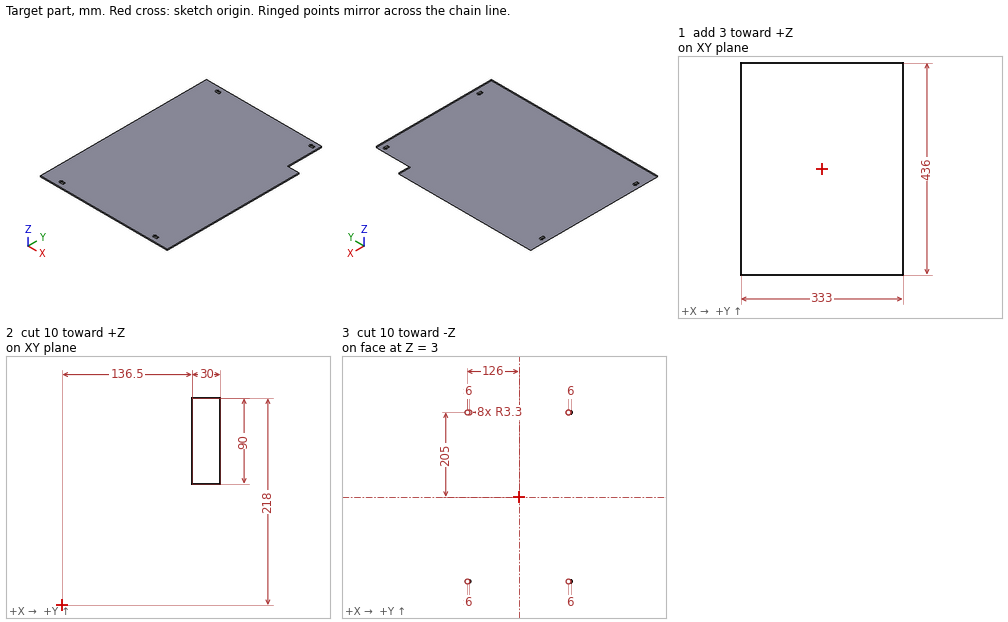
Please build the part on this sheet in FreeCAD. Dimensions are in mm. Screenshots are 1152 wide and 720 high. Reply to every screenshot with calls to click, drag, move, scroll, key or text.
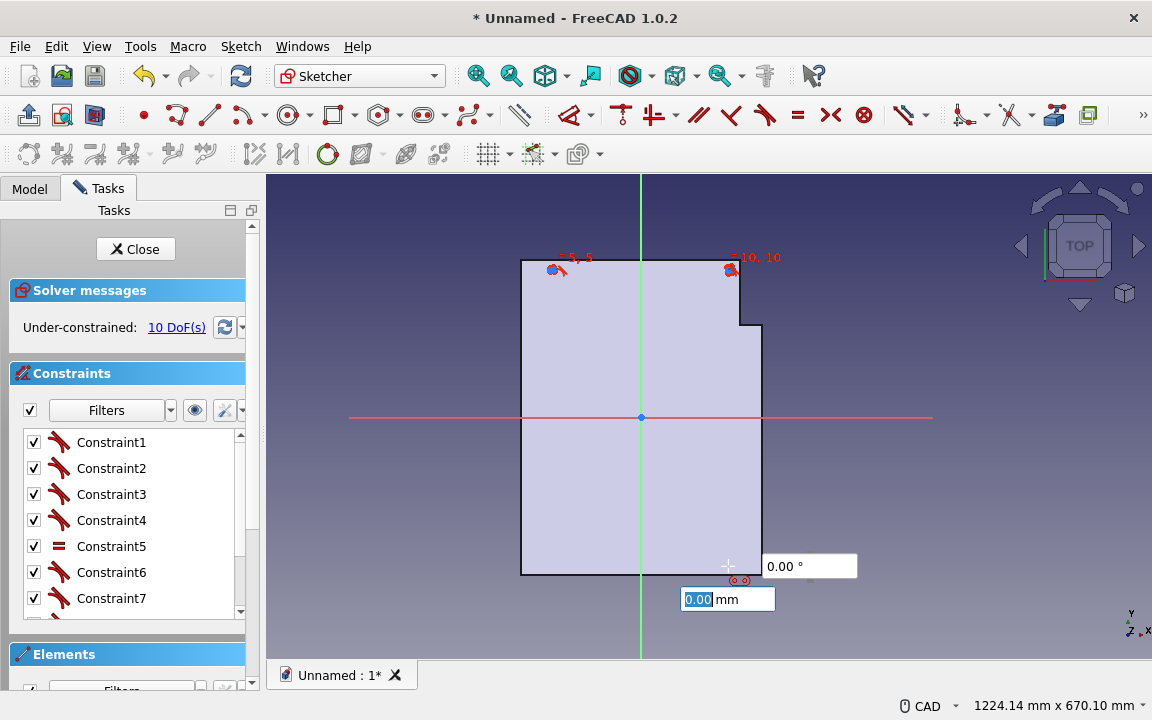
scroll(732, 566, up, 7)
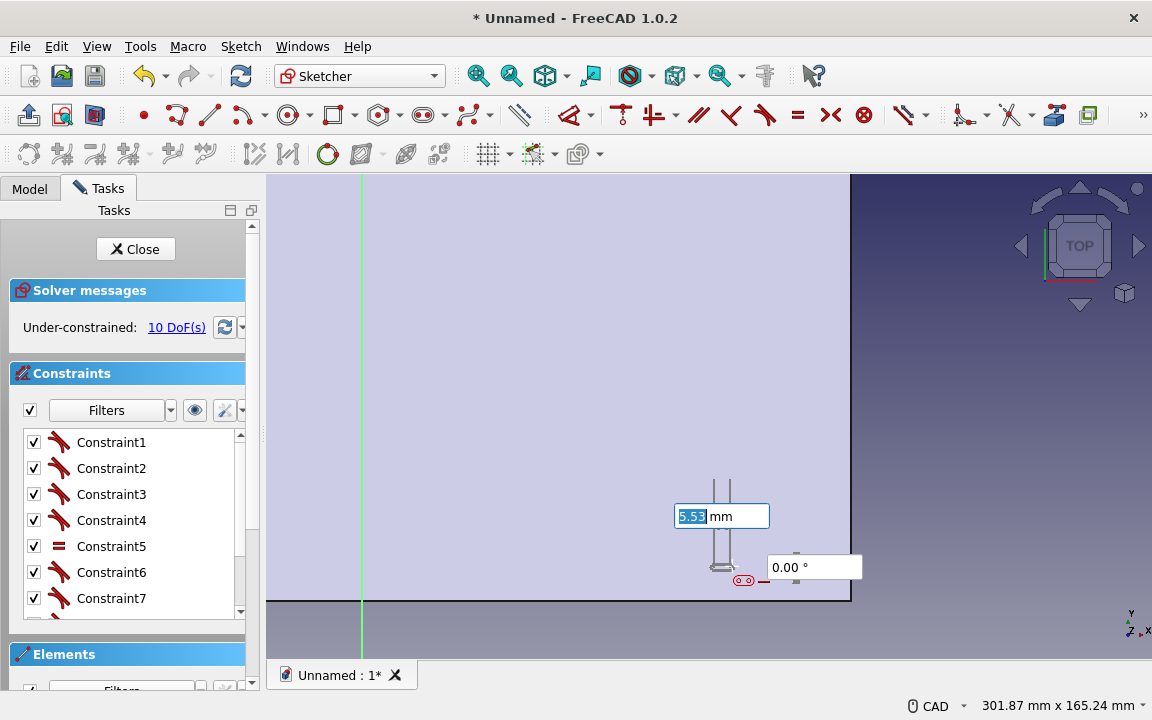
click(732, 564)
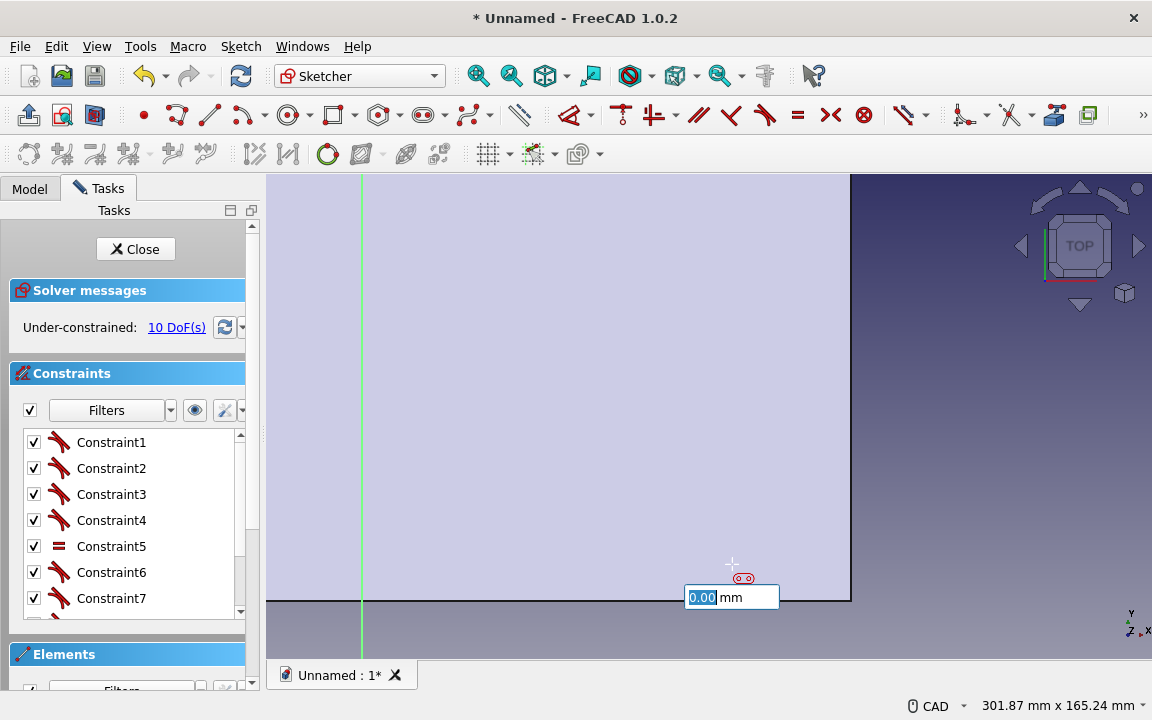
scroll(723, 554, up, 3)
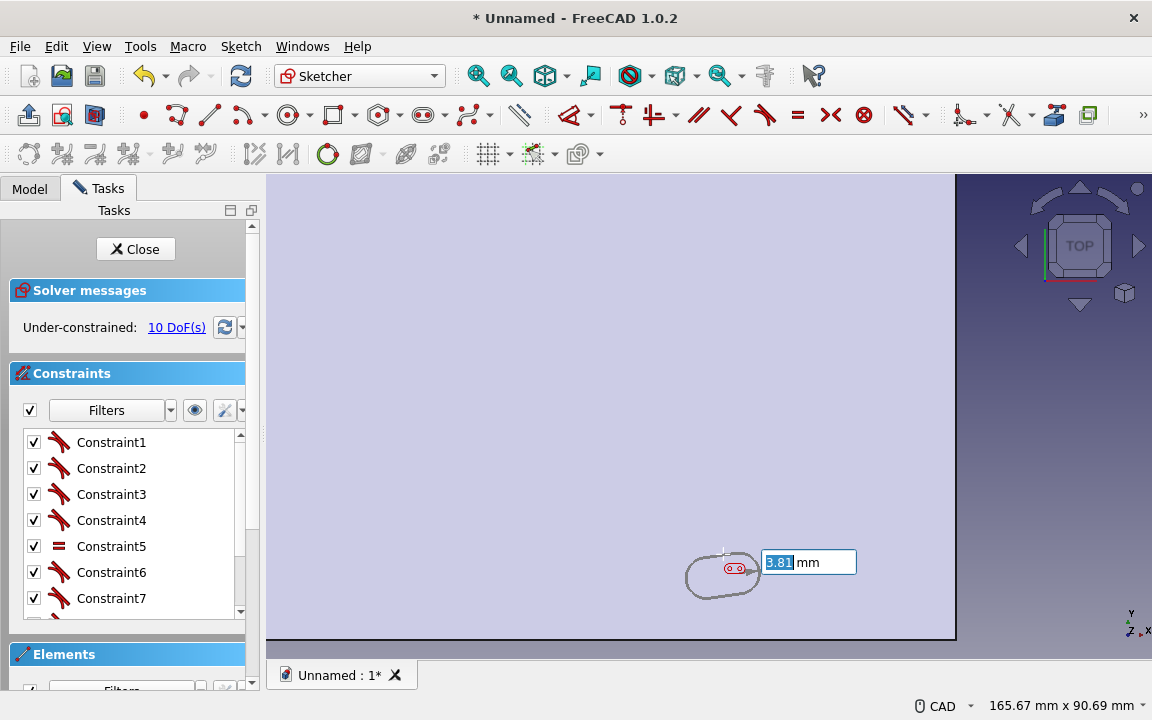
click(723, 553)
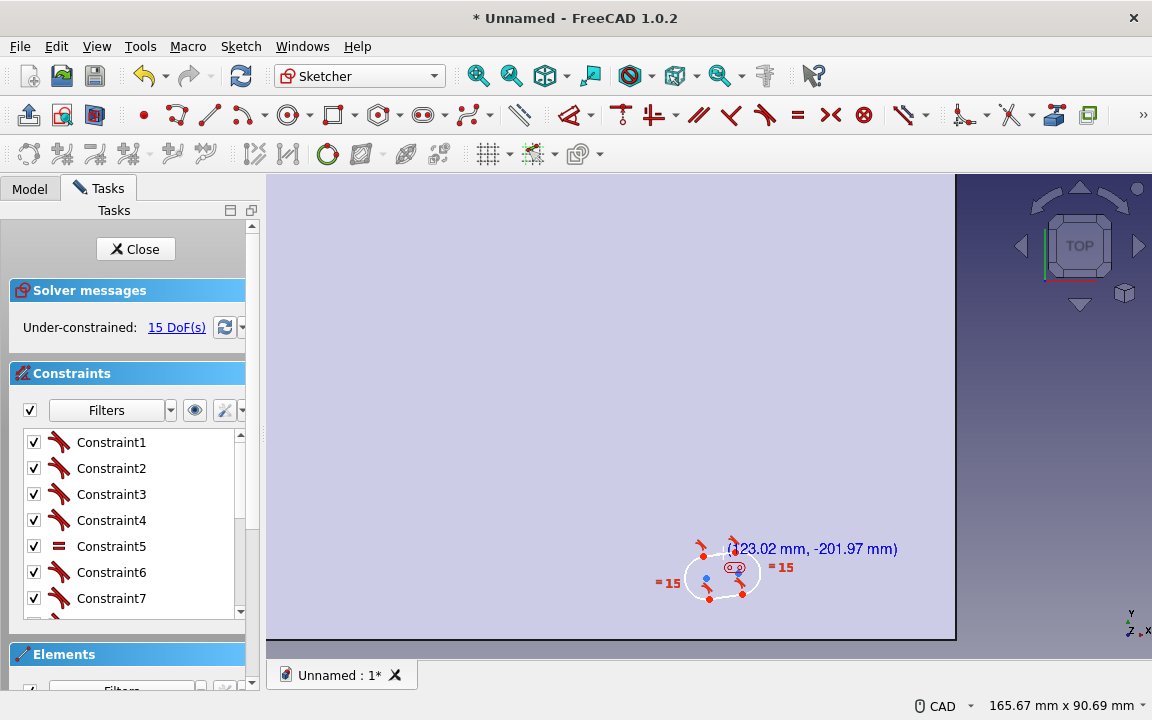
scroll(731, 564, down, 10)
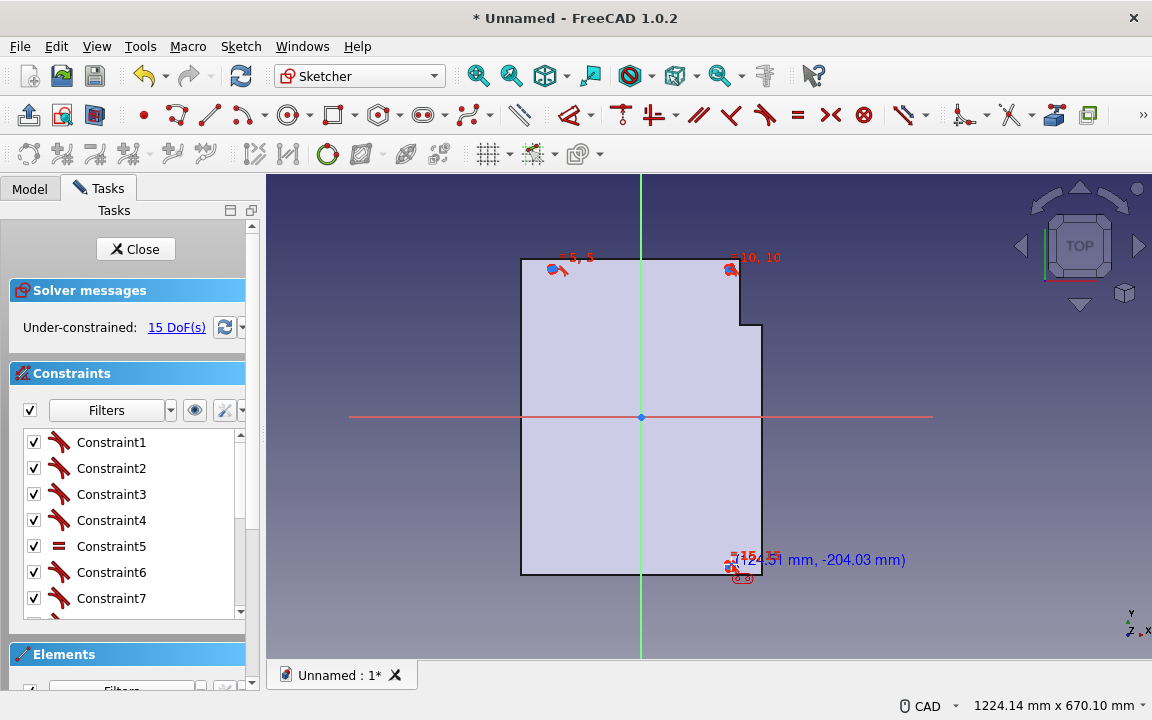
scroll(550, 566, up, 12)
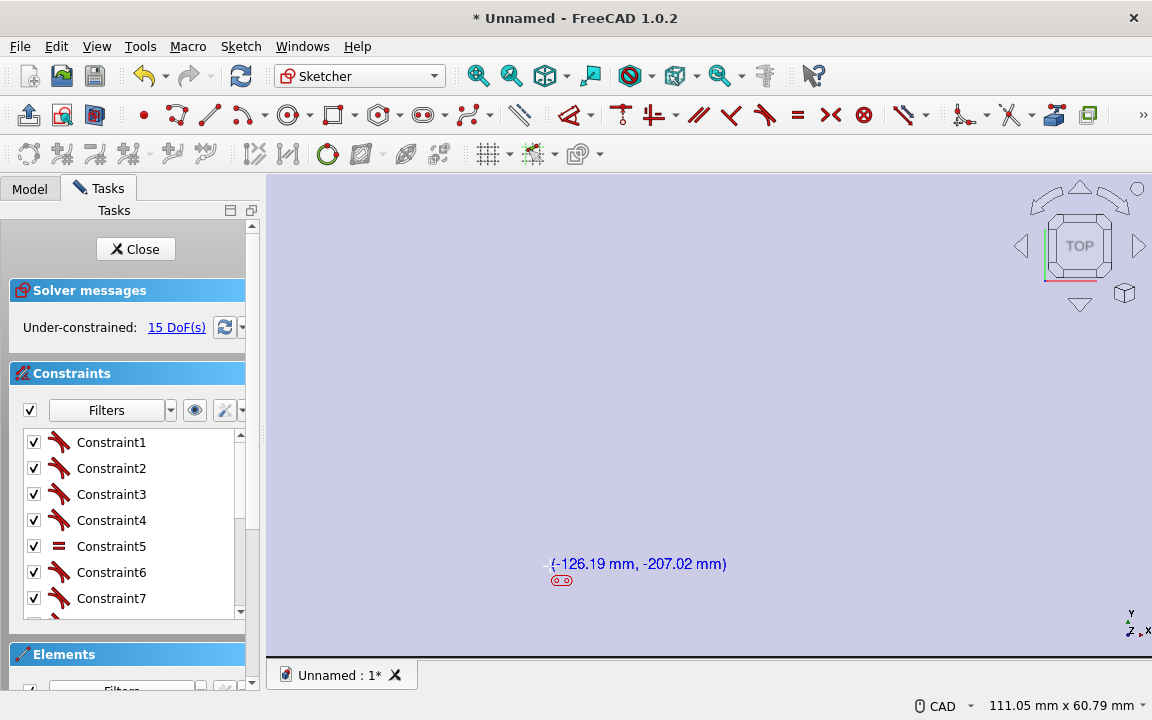
scroll(549, 566, down, 12)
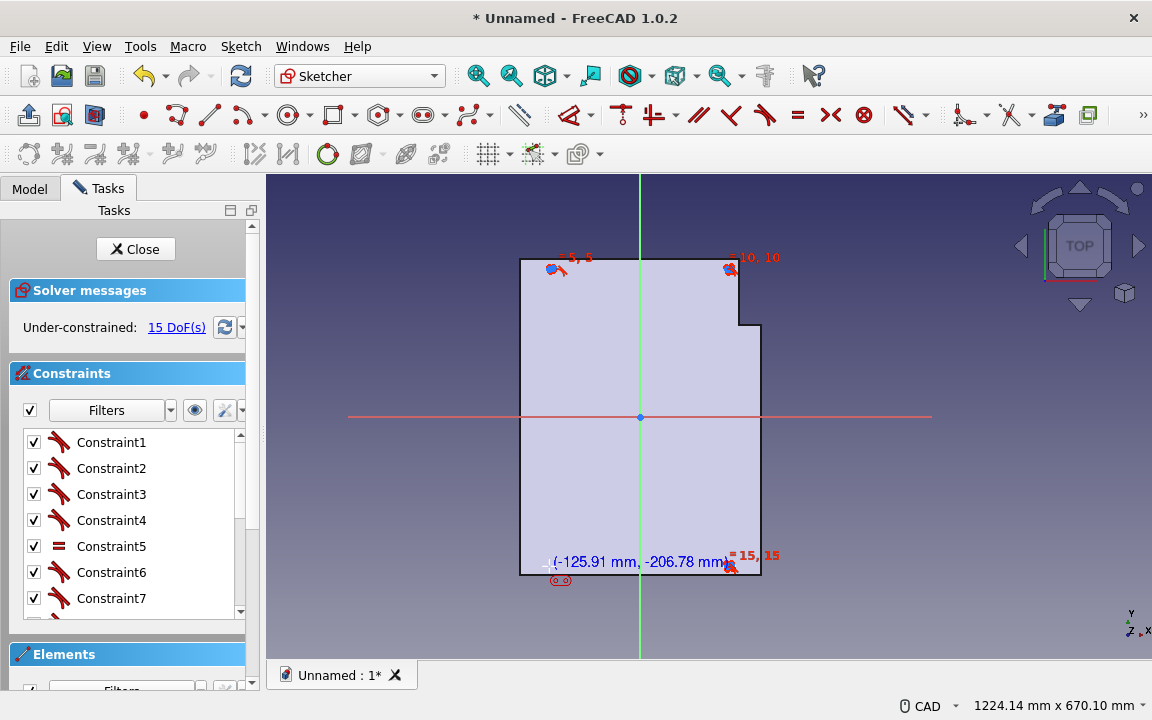
click(549, 566)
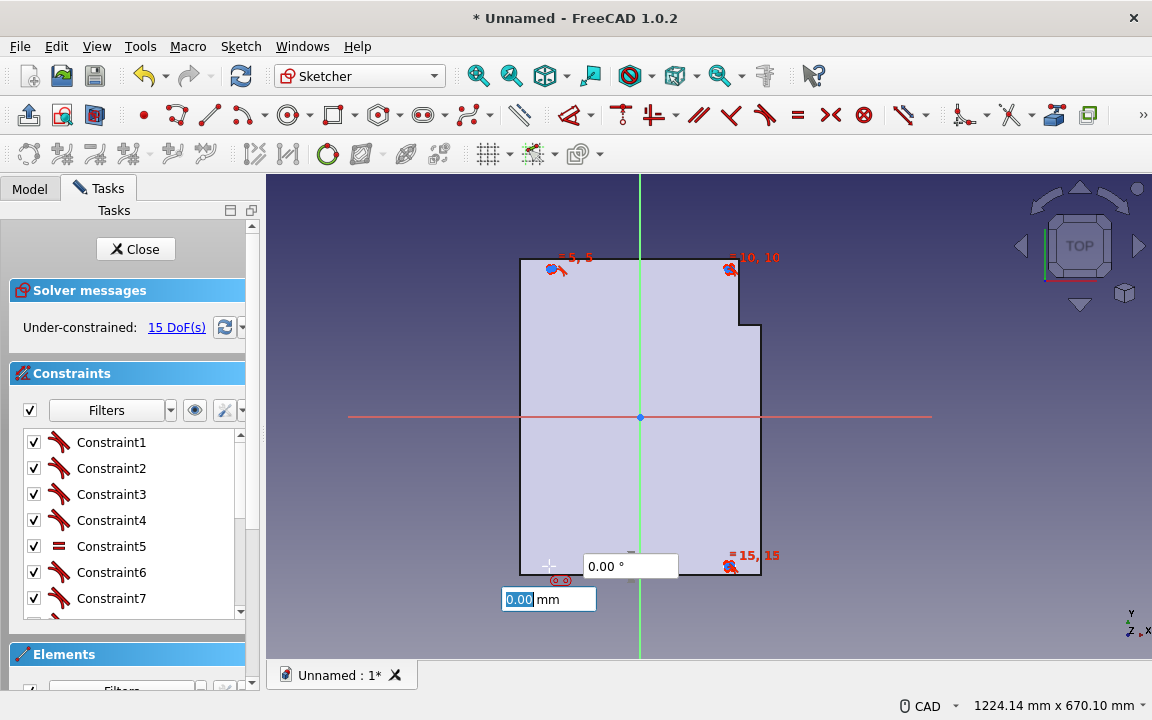
scroll(554, 566, up, 7)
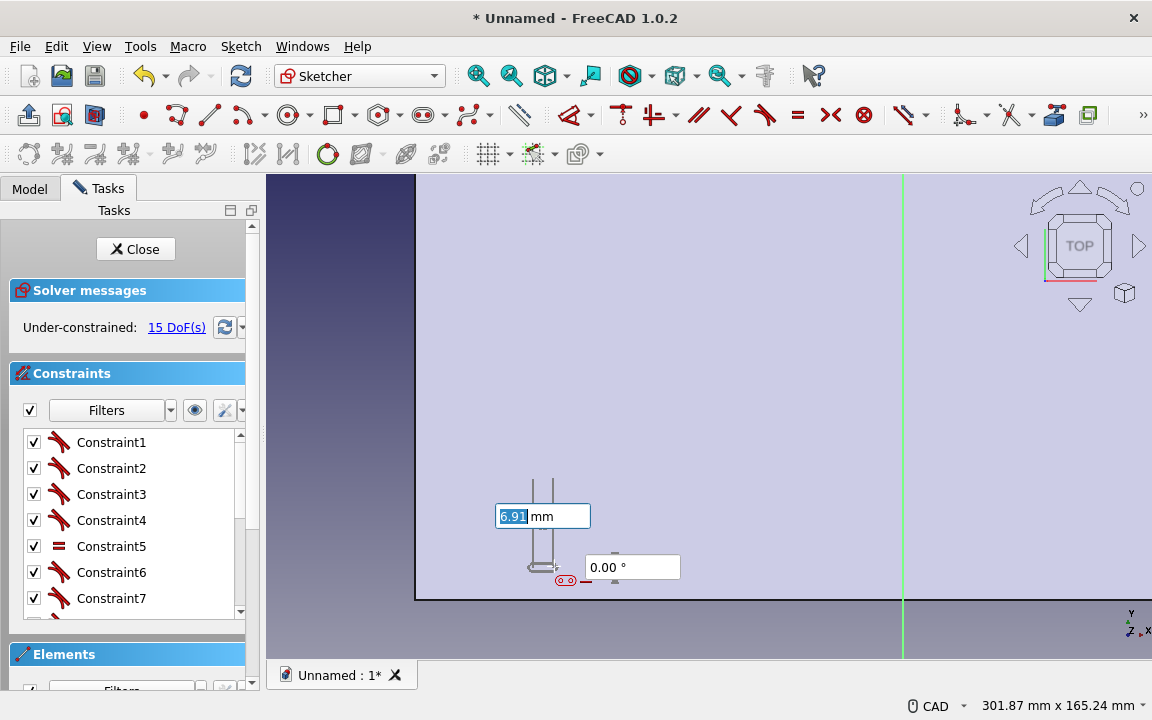
click(551, 564)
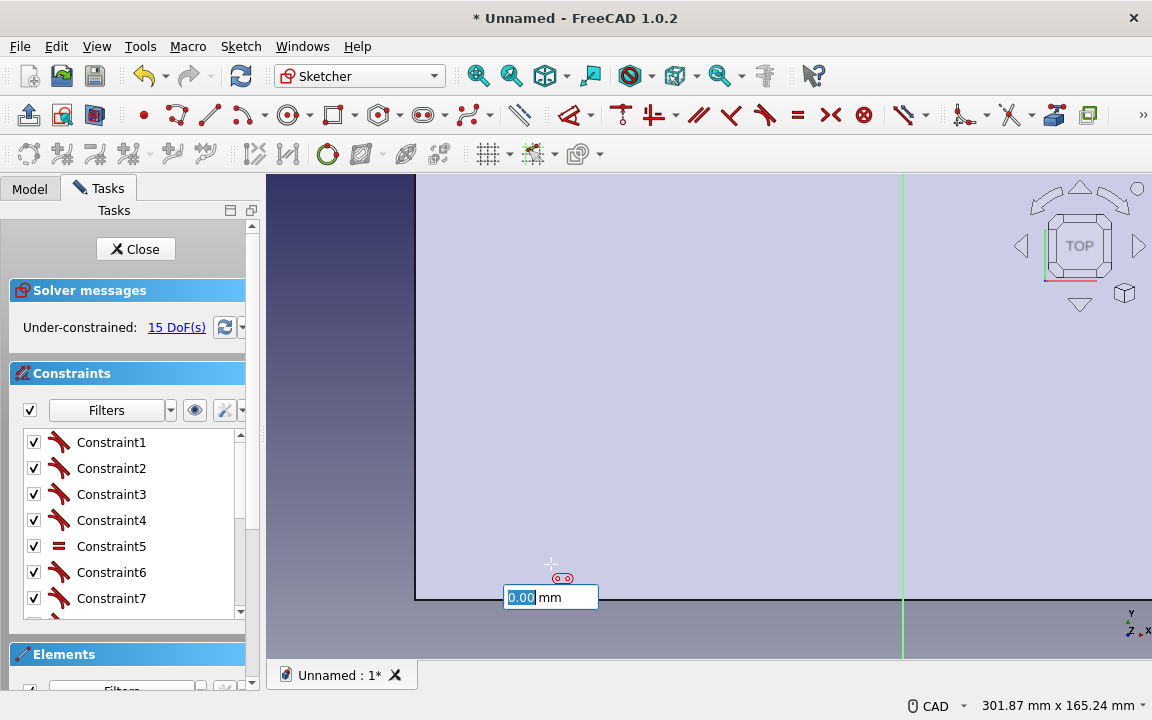
scroll(542, 571, up, 3)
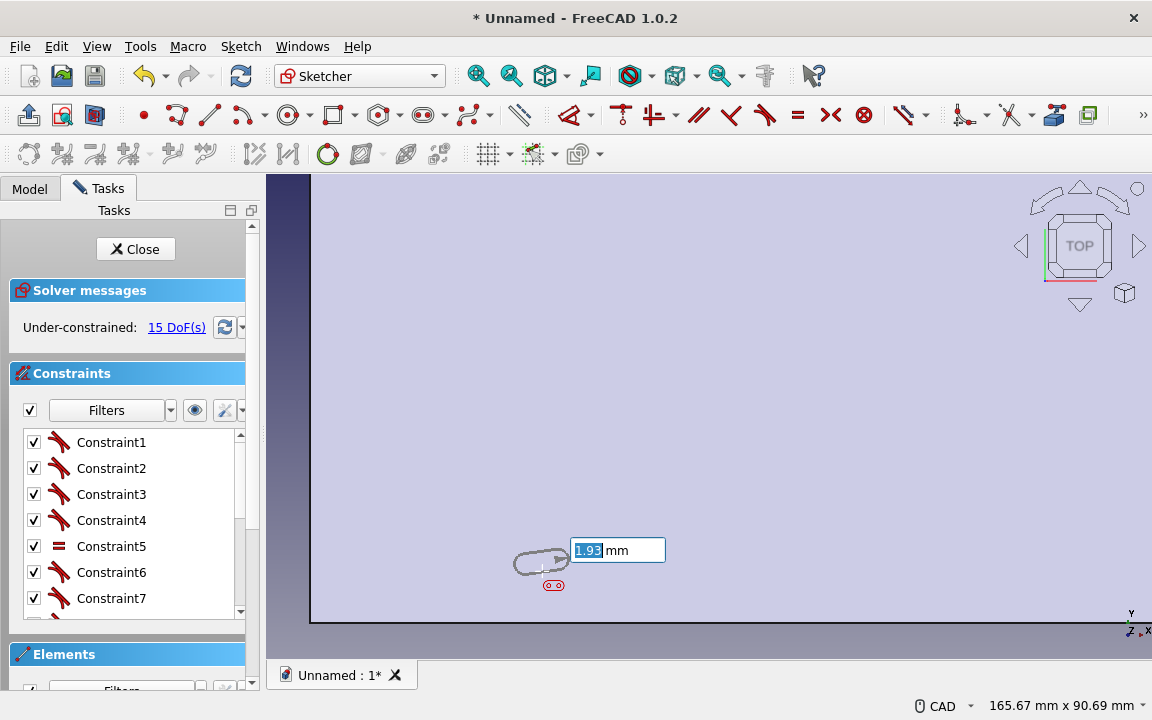
click(543, 571)
key(Escape)